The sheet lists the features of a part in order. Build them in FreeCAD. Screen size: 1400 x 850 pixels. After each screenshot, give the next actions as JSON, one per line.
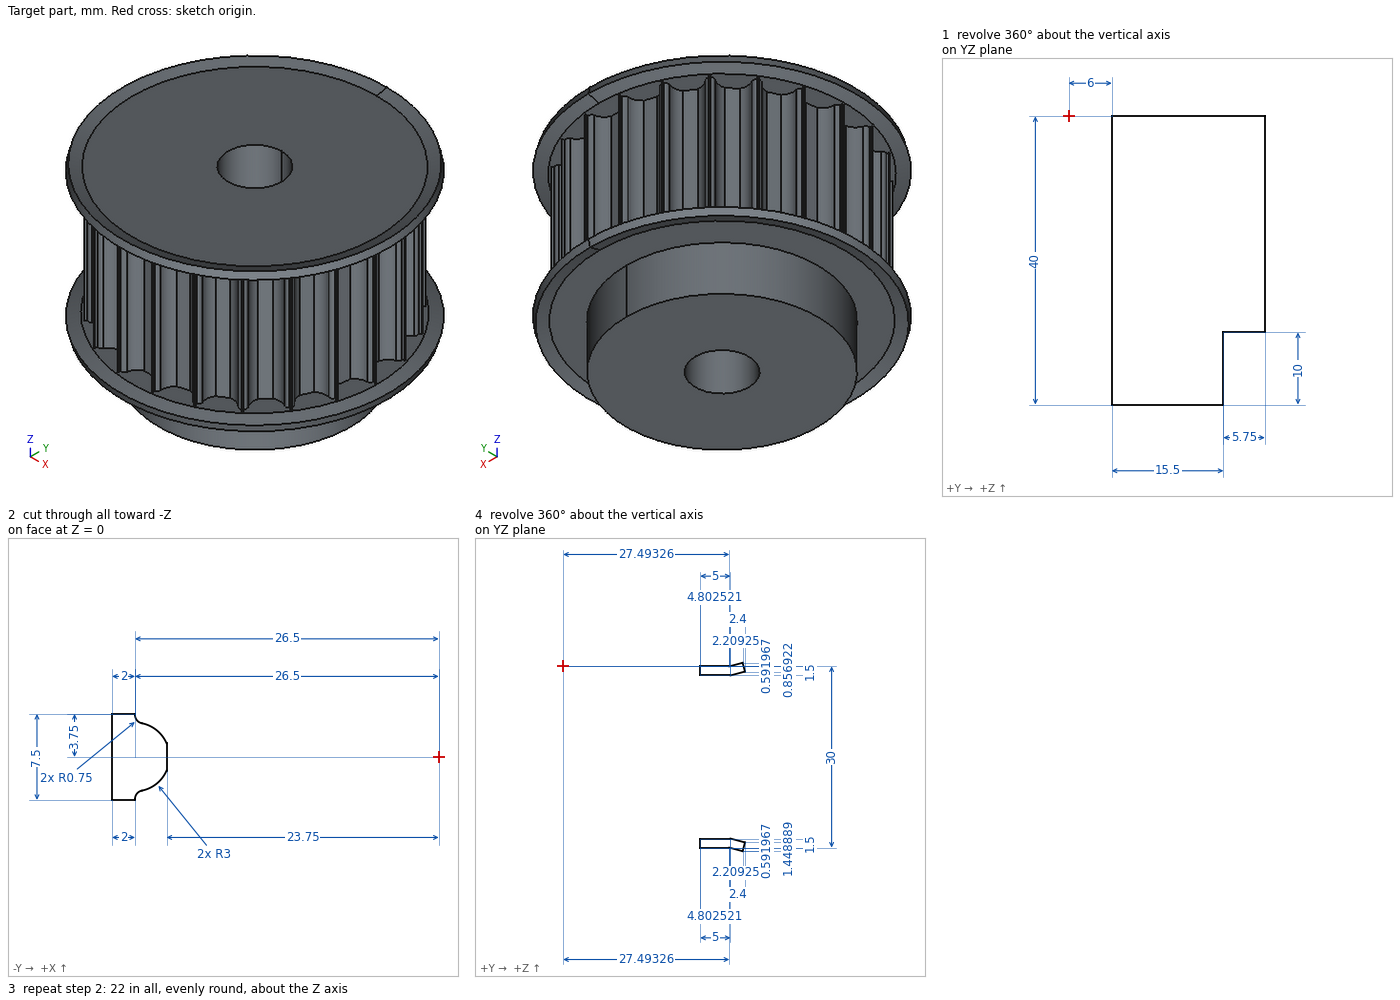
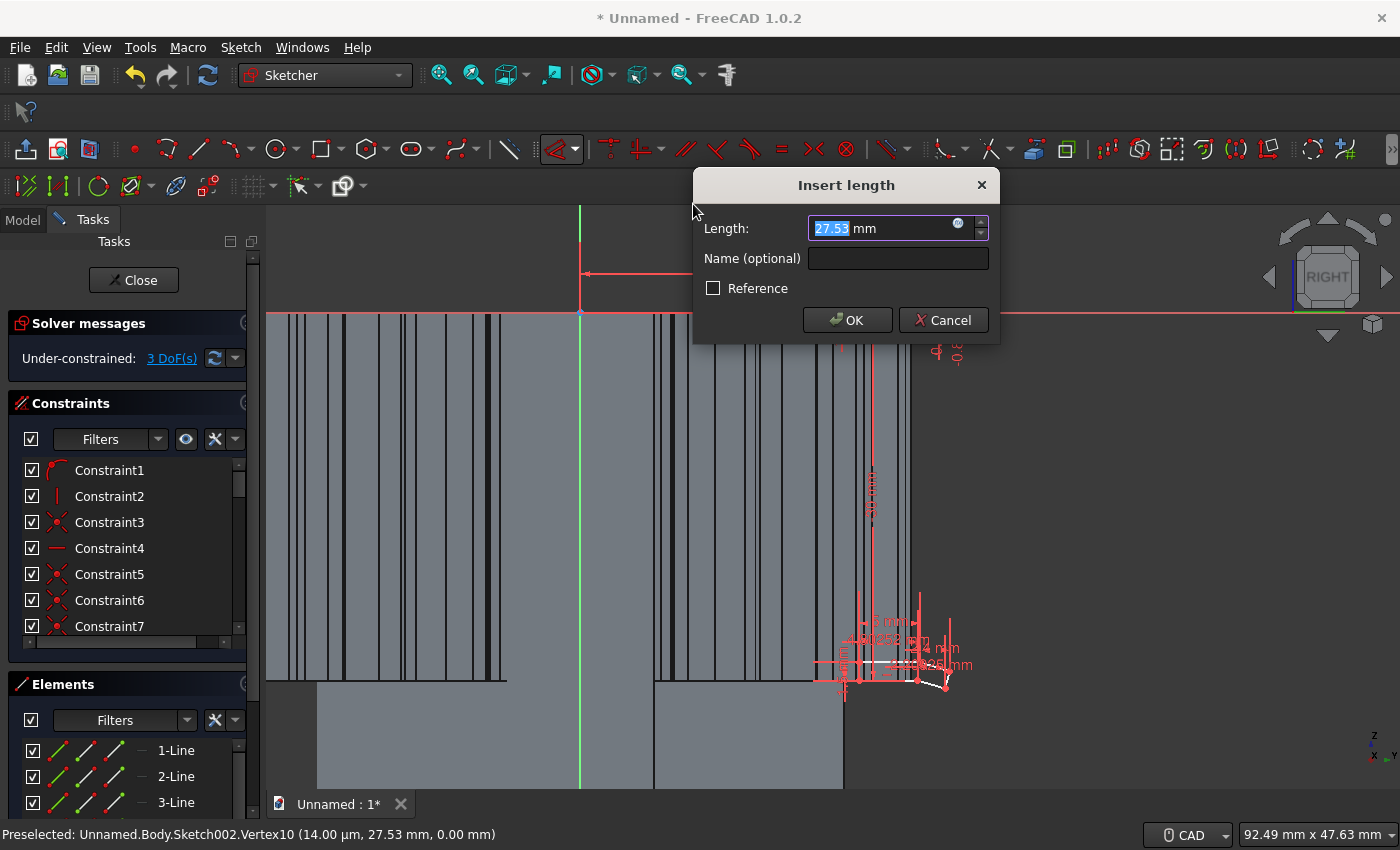
{"action": "type", "text": "27.49326"}
{"action": "key", "text": "Return"}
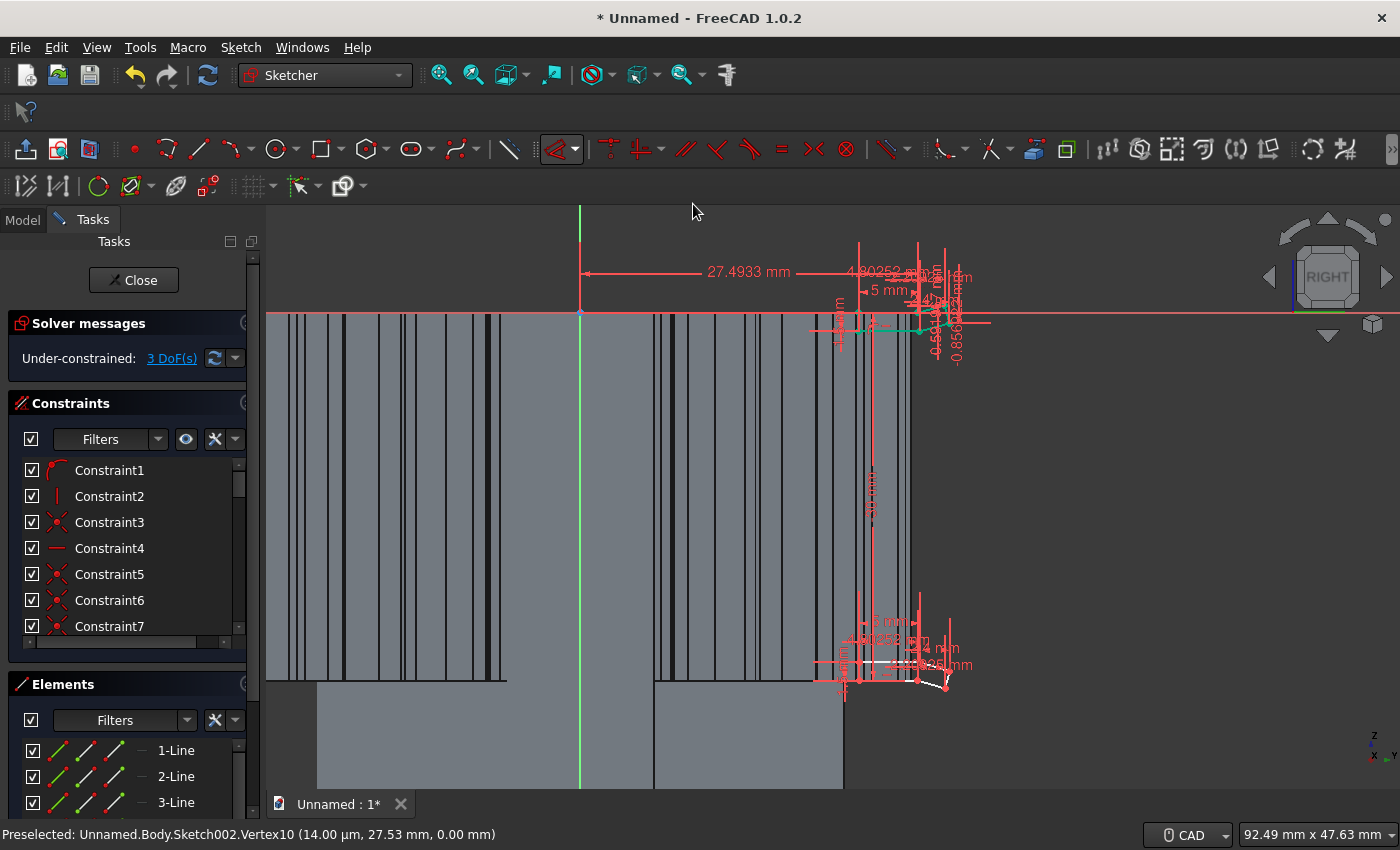
{"action": "left_click", "coordinate": [918, 681]}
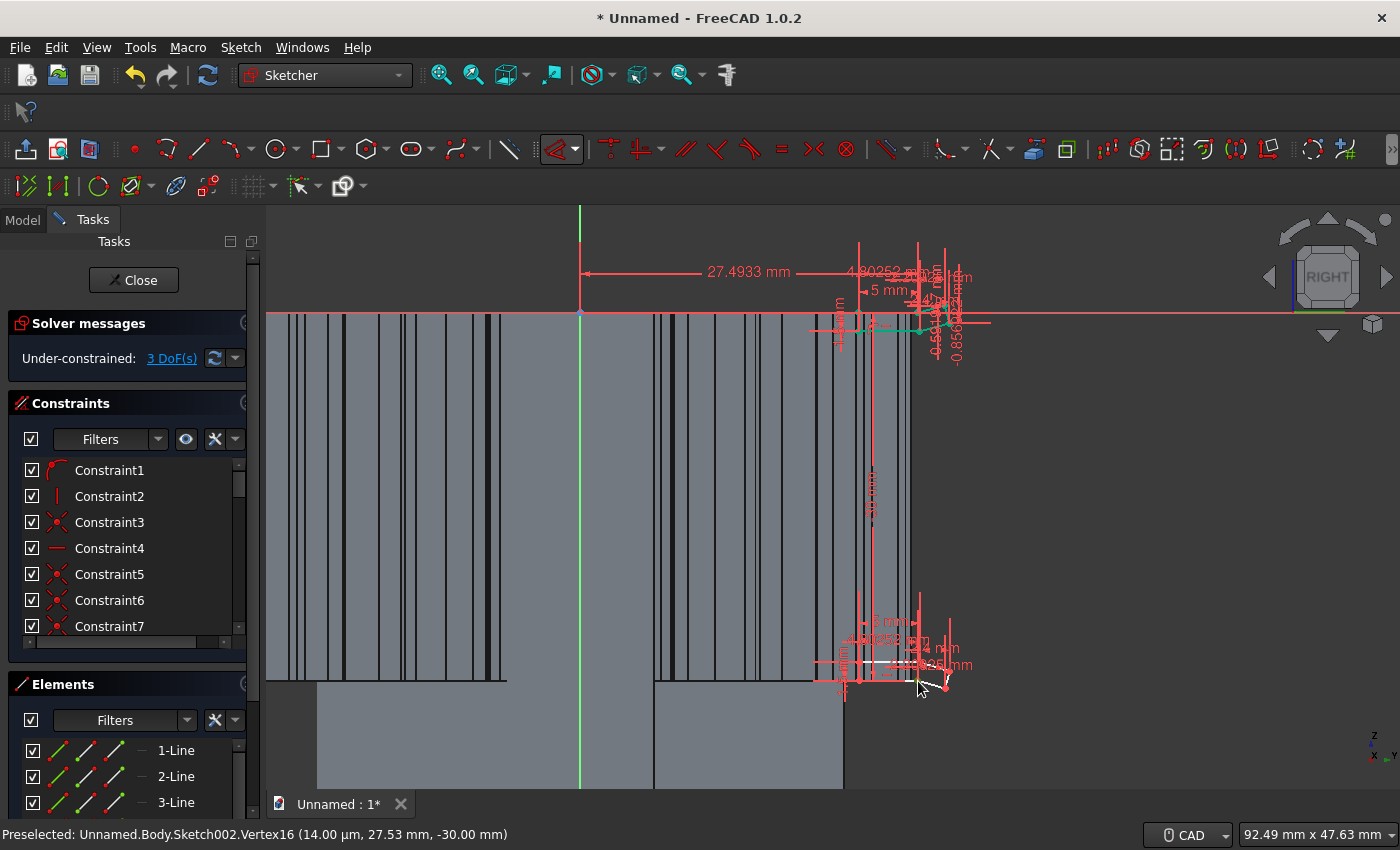
{"action": "left_click", "coordinate": [578, 150]}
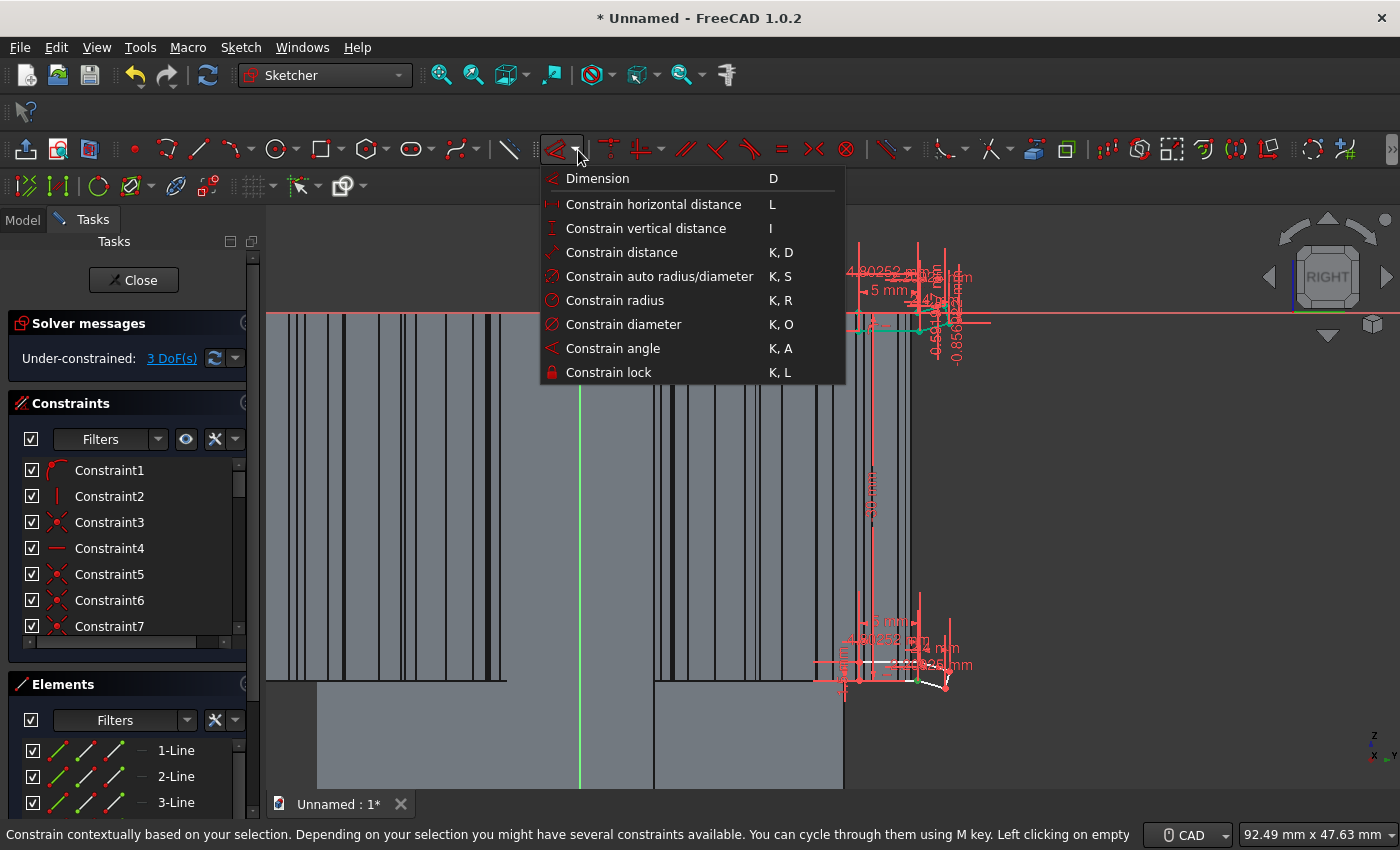
{"action": "left_click", "coordinate": [693, 204]}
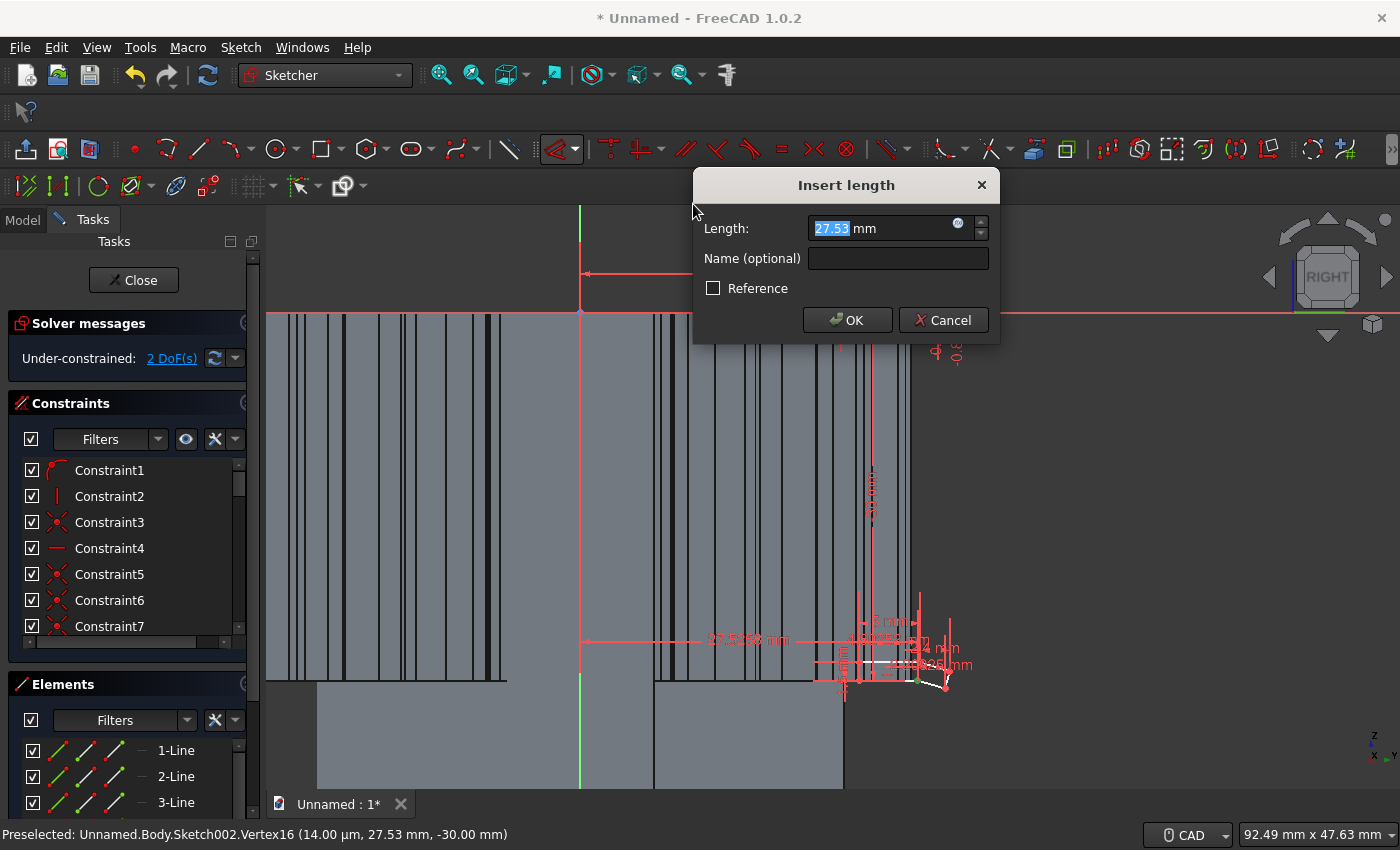
{"action": "type", "text": "27.49326"}
{"action": "key", "text": "Return"}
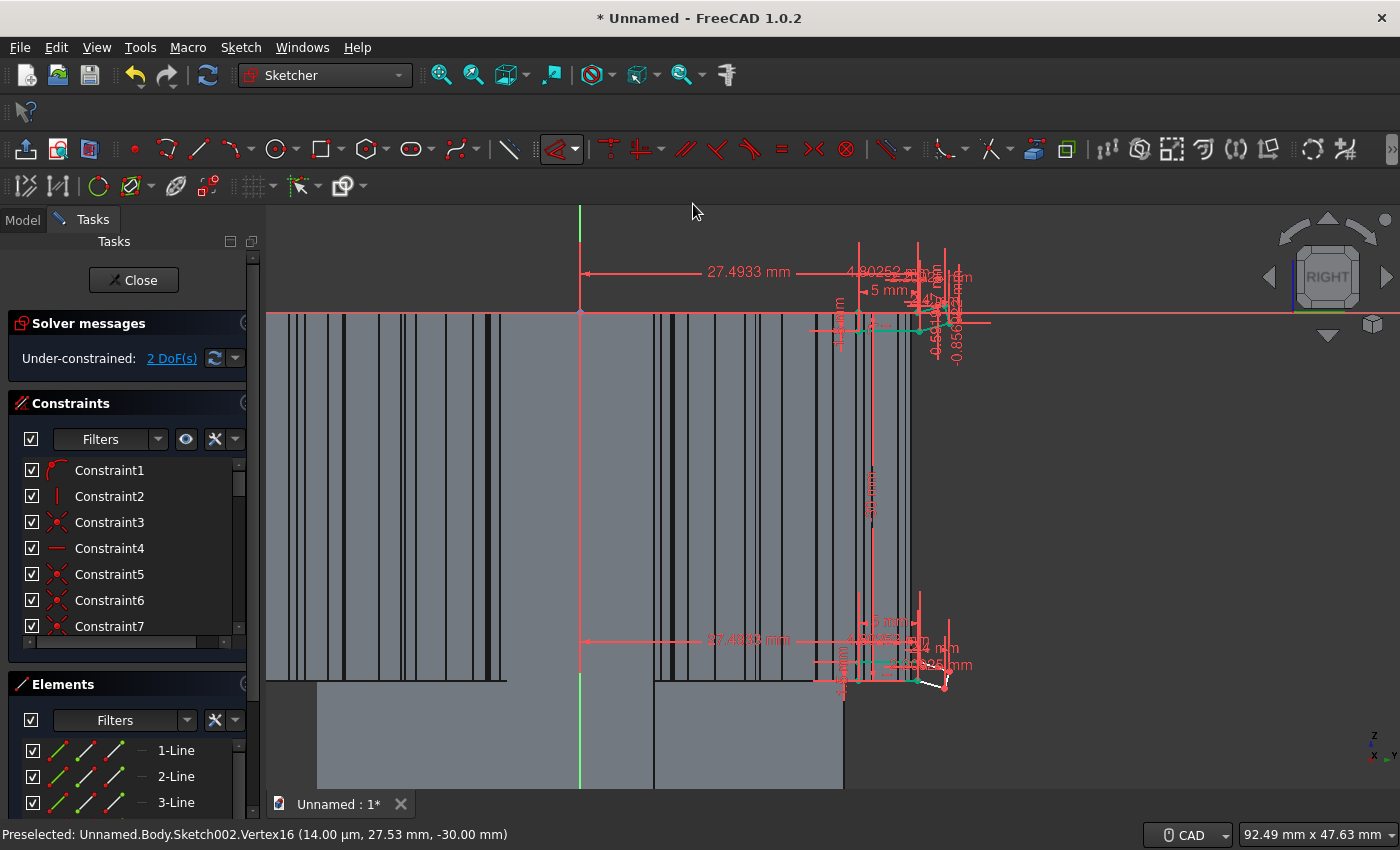
{"action": "scroll", "coordinate": [928, 684], "scroll_direction": "up", "scroll_amount": 9}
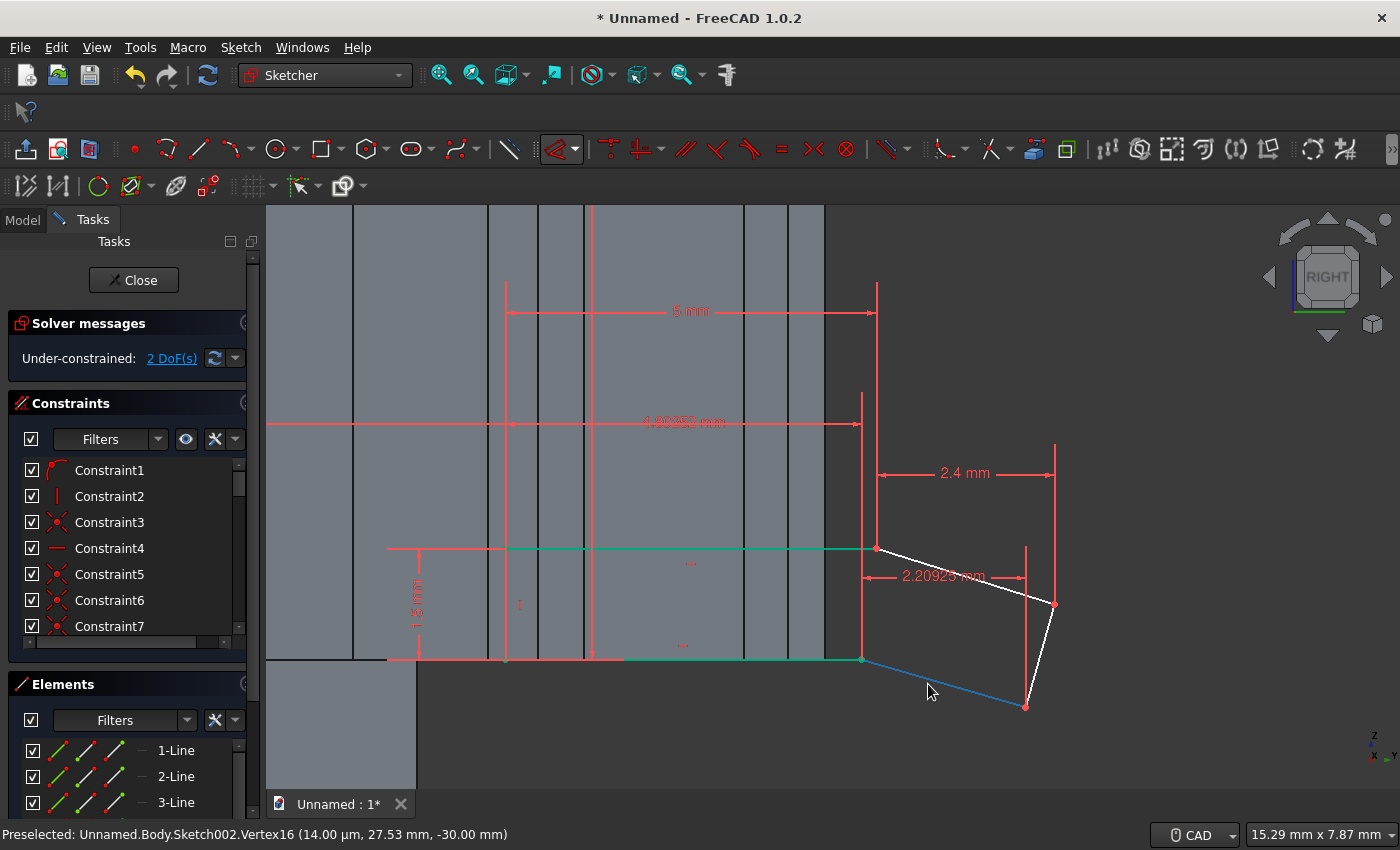
{"action": "left_click", "coordinate": [927, 679]}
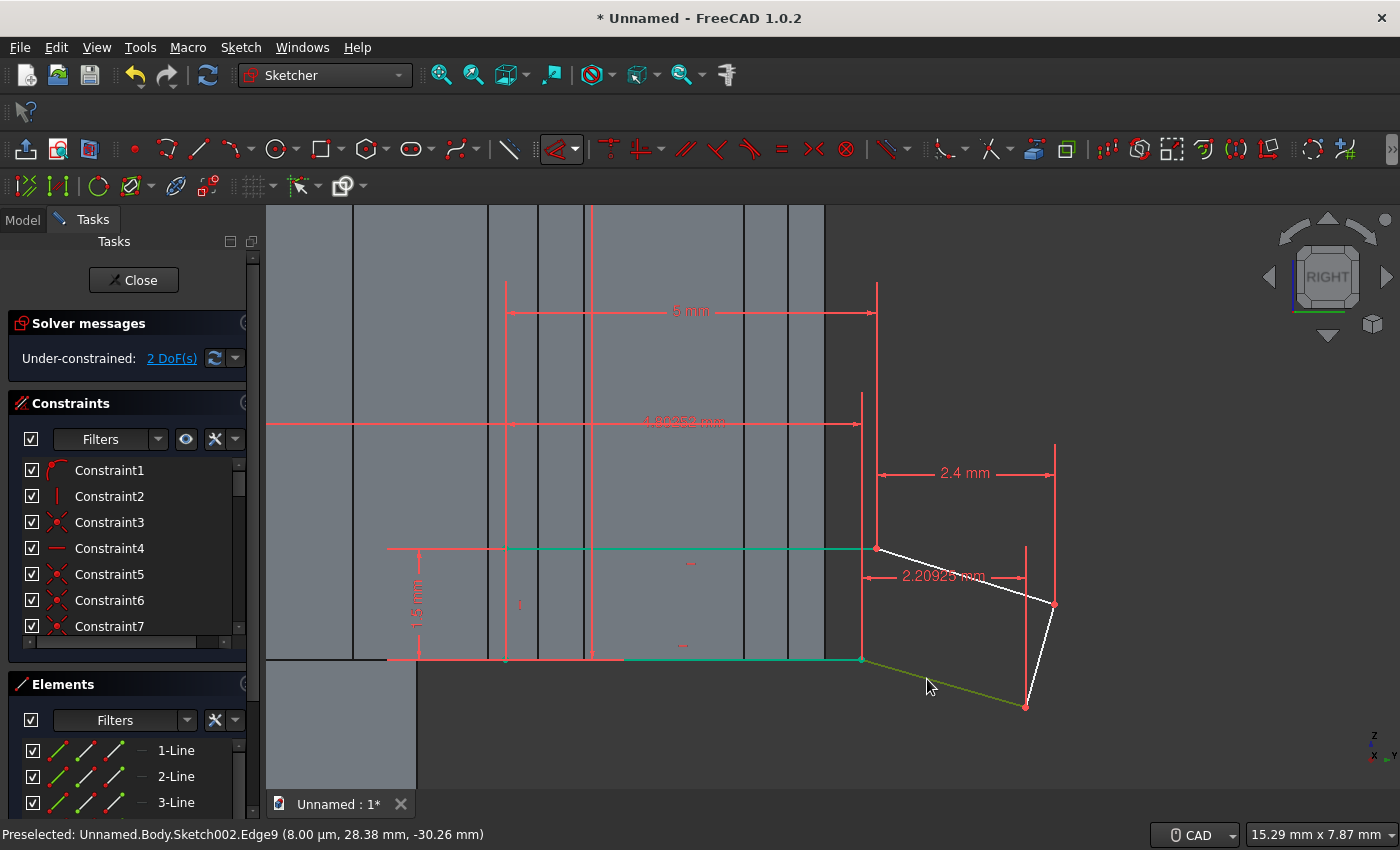
{"action": "left_click", "coordinate": [578, 150]}